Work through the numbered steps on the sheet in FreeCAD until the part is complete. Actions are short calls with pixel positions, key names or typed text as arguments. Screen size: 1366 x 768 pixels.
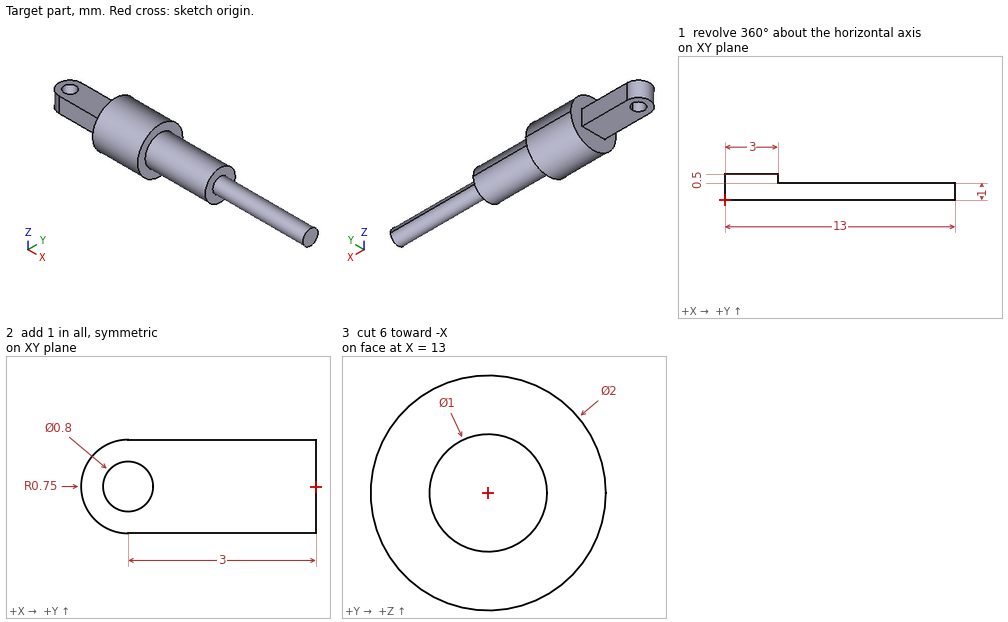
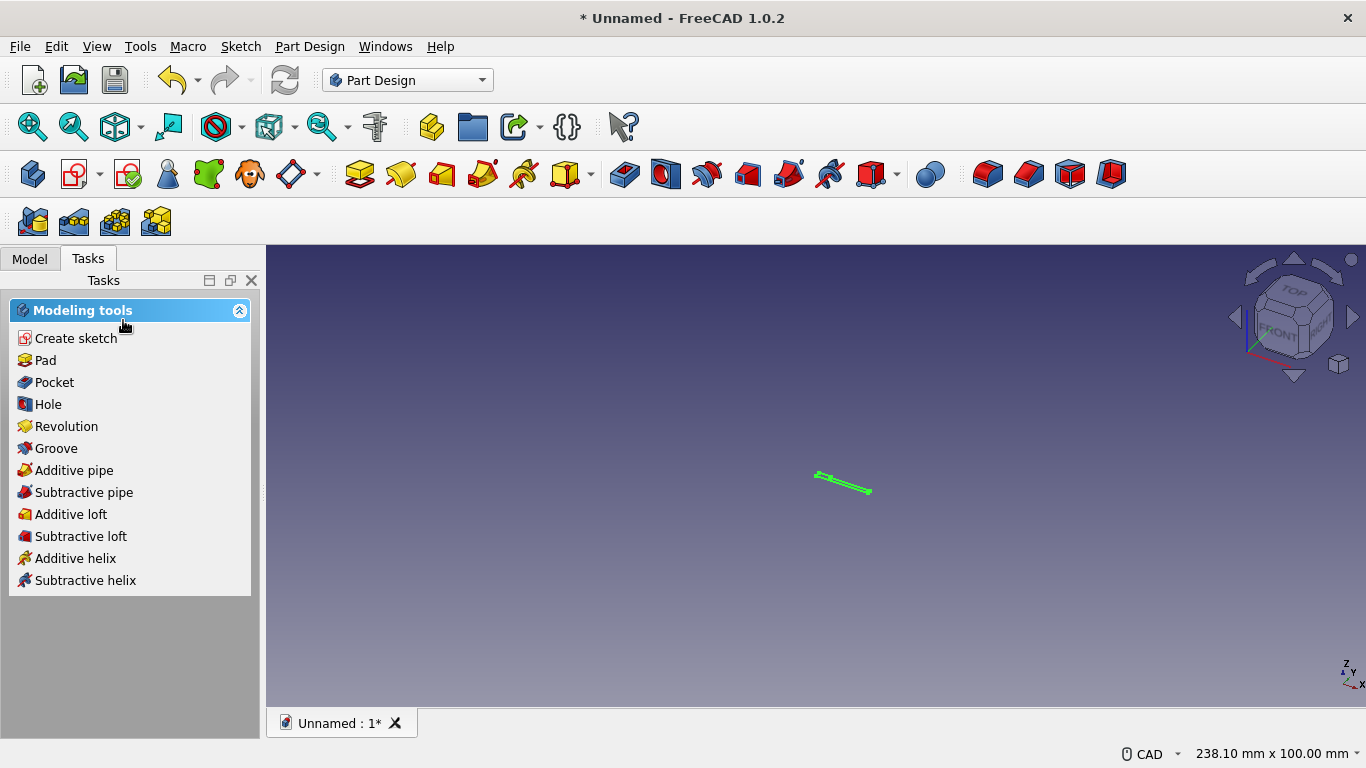
click(401, 174)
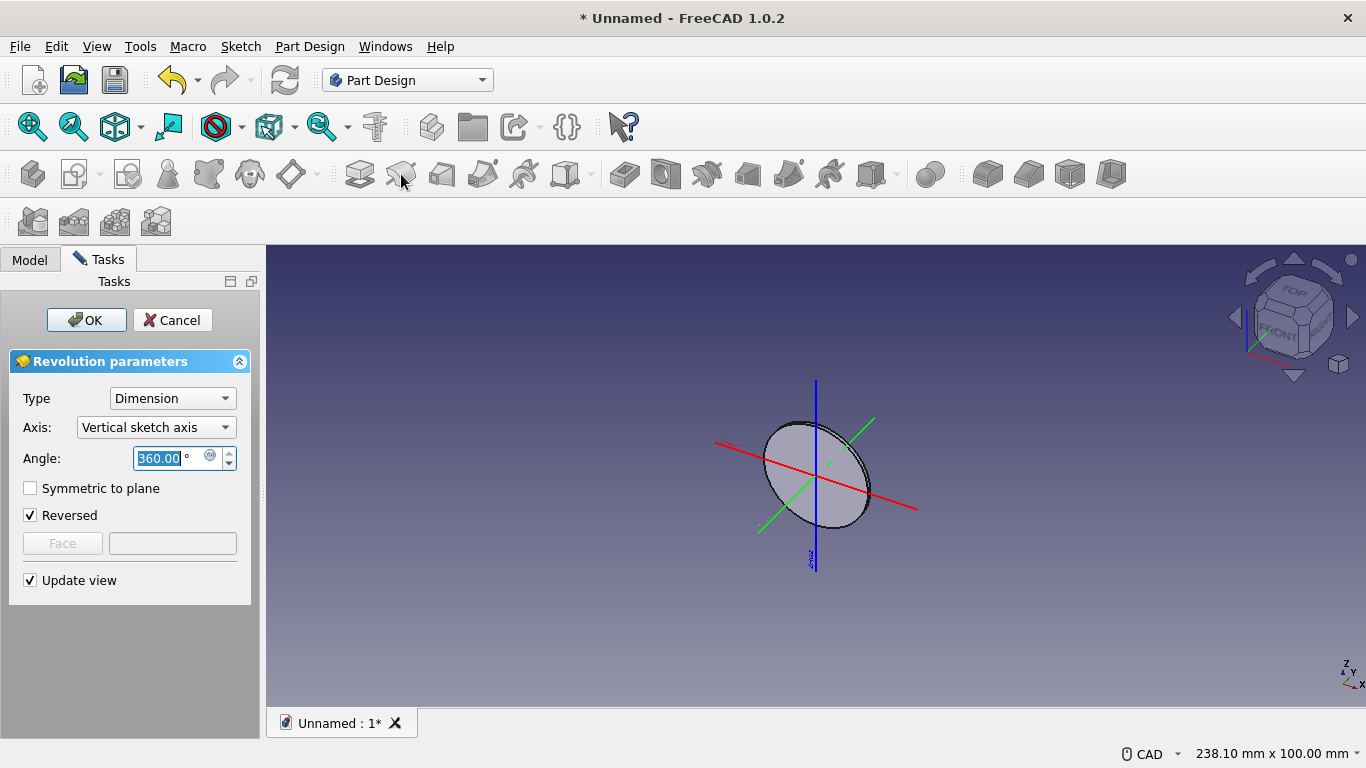
click(157, 428)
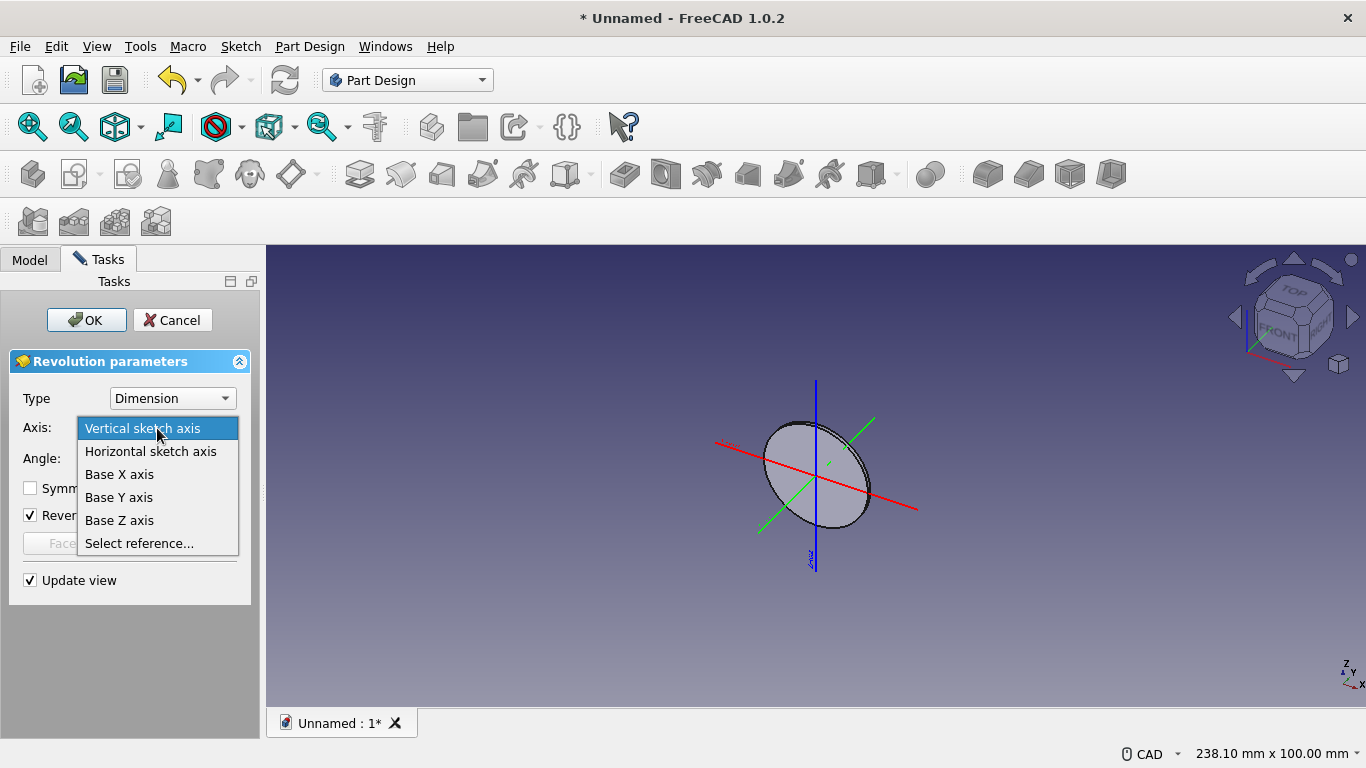
click(156, 452)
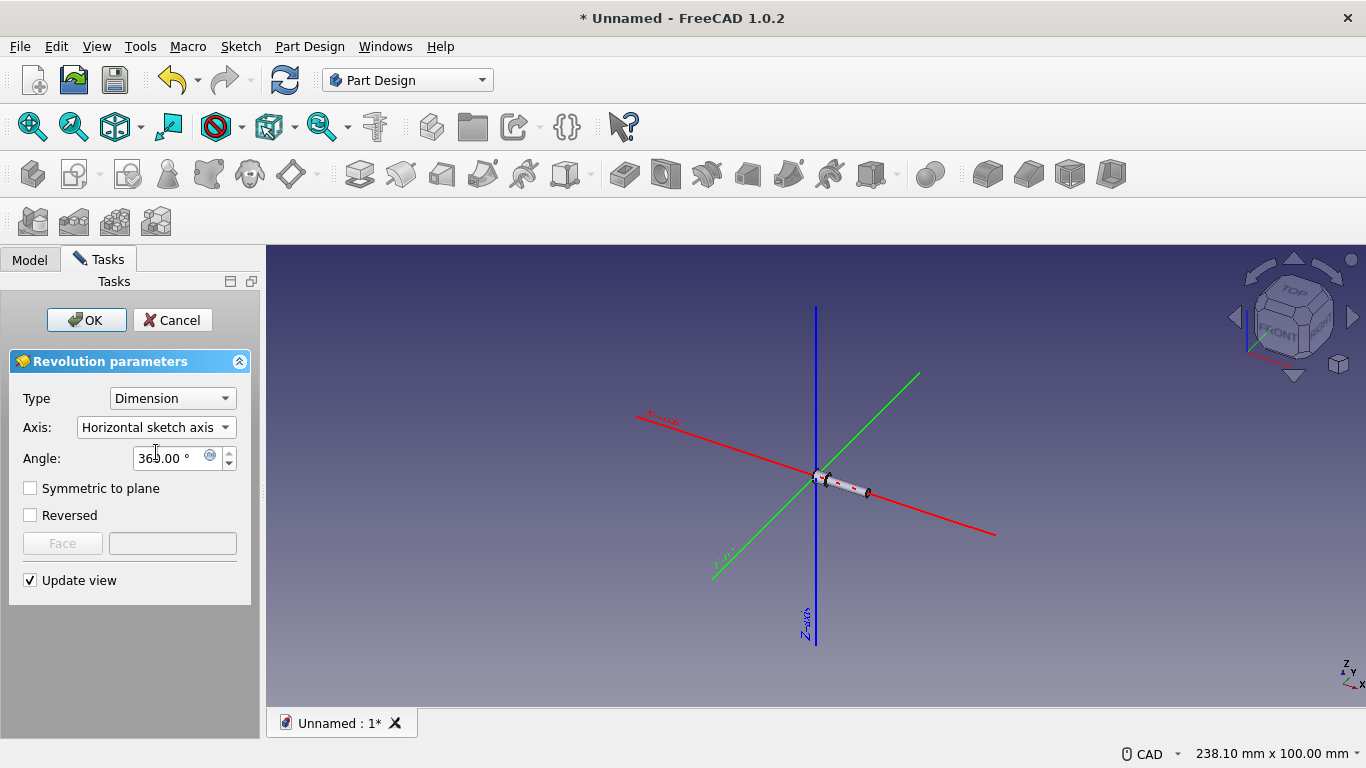
click(87, 320)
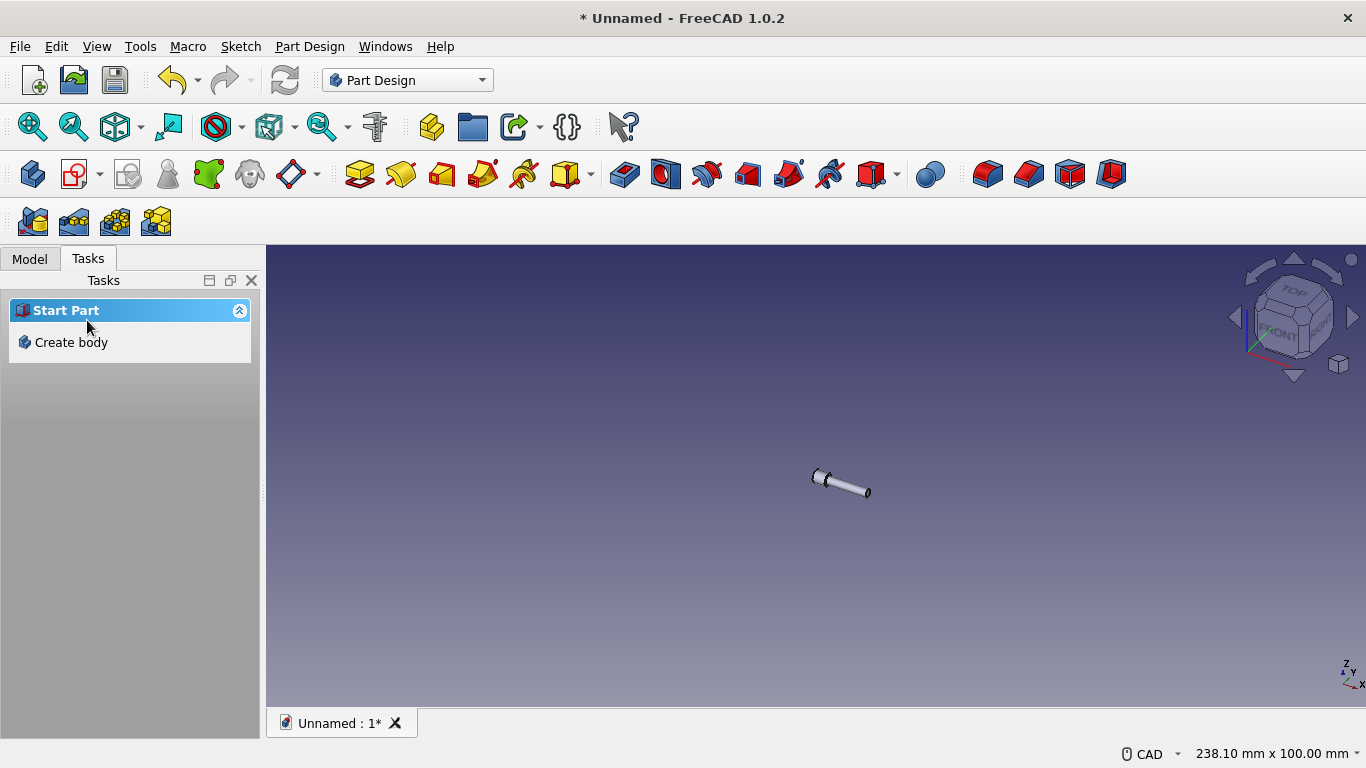
click(33, 128)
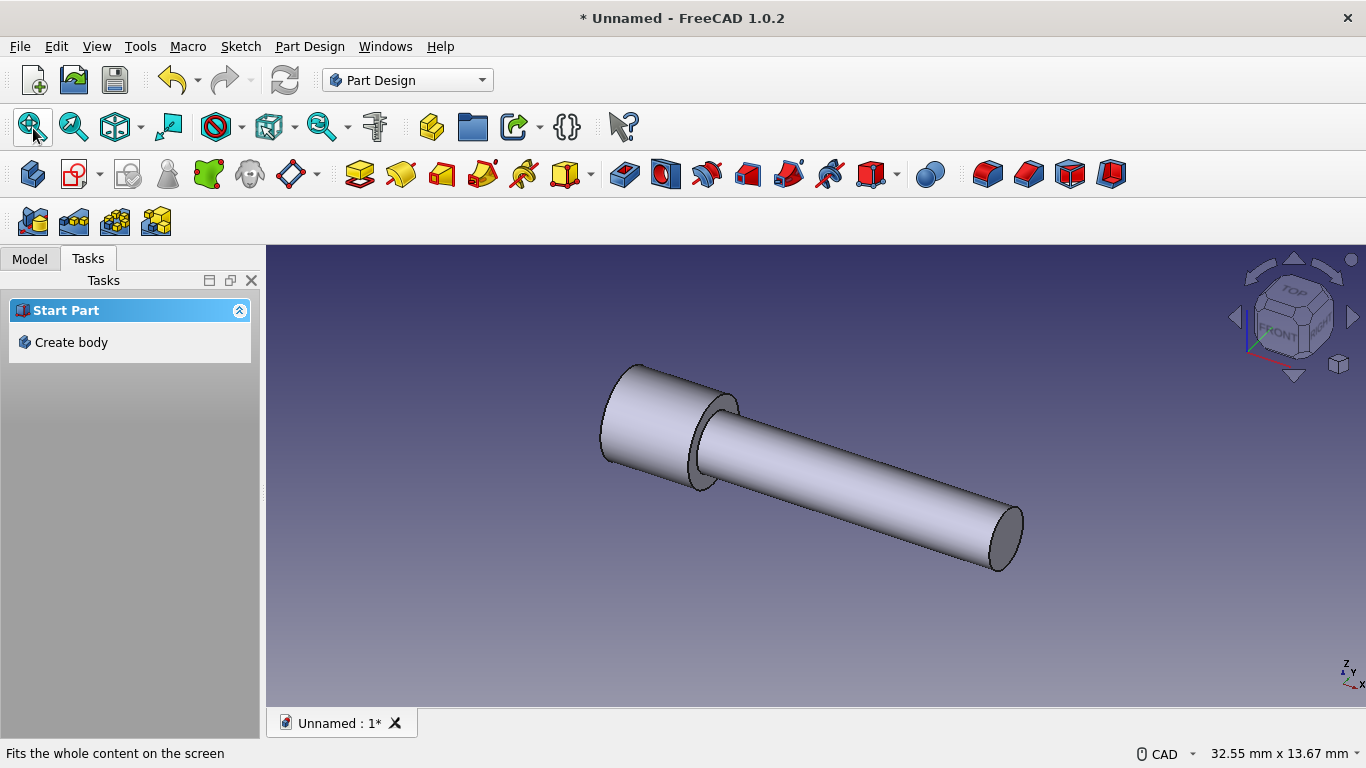
click(74, 174)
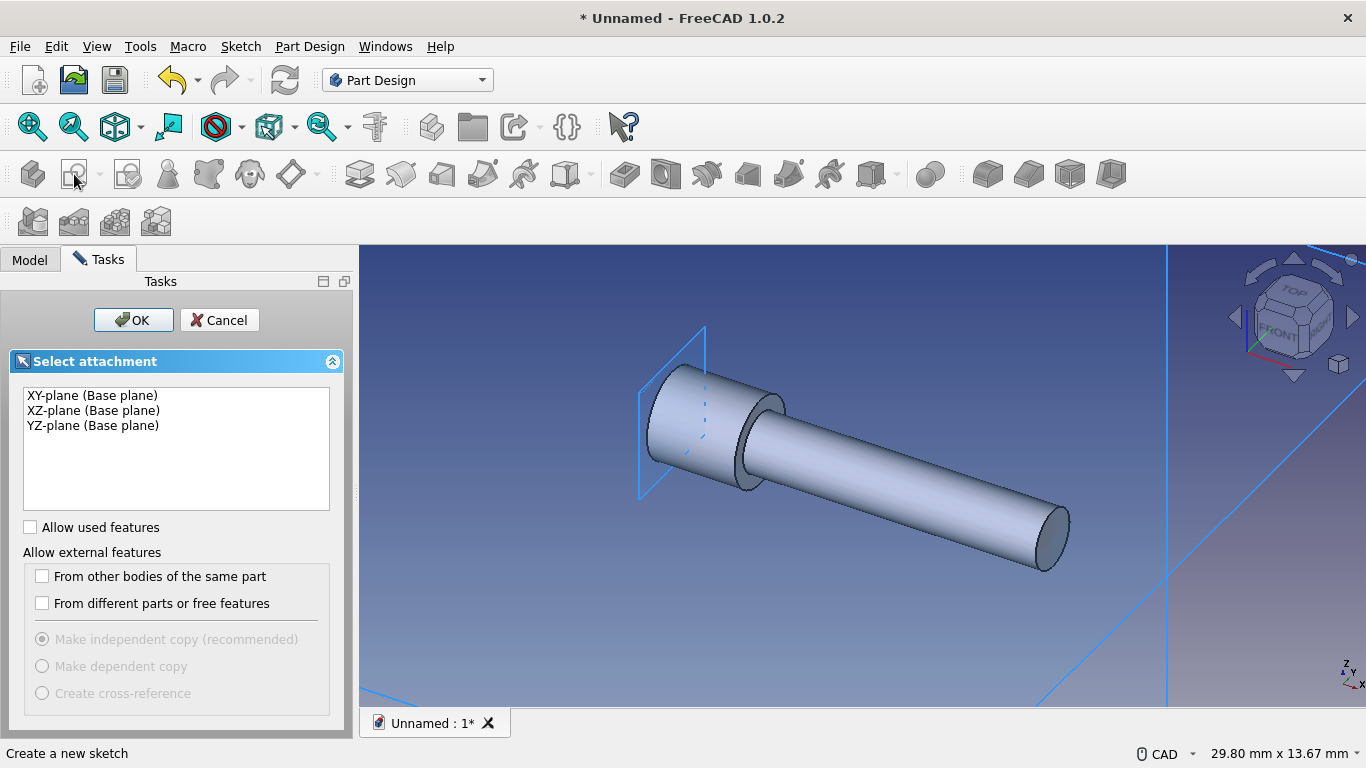
click(84, 396)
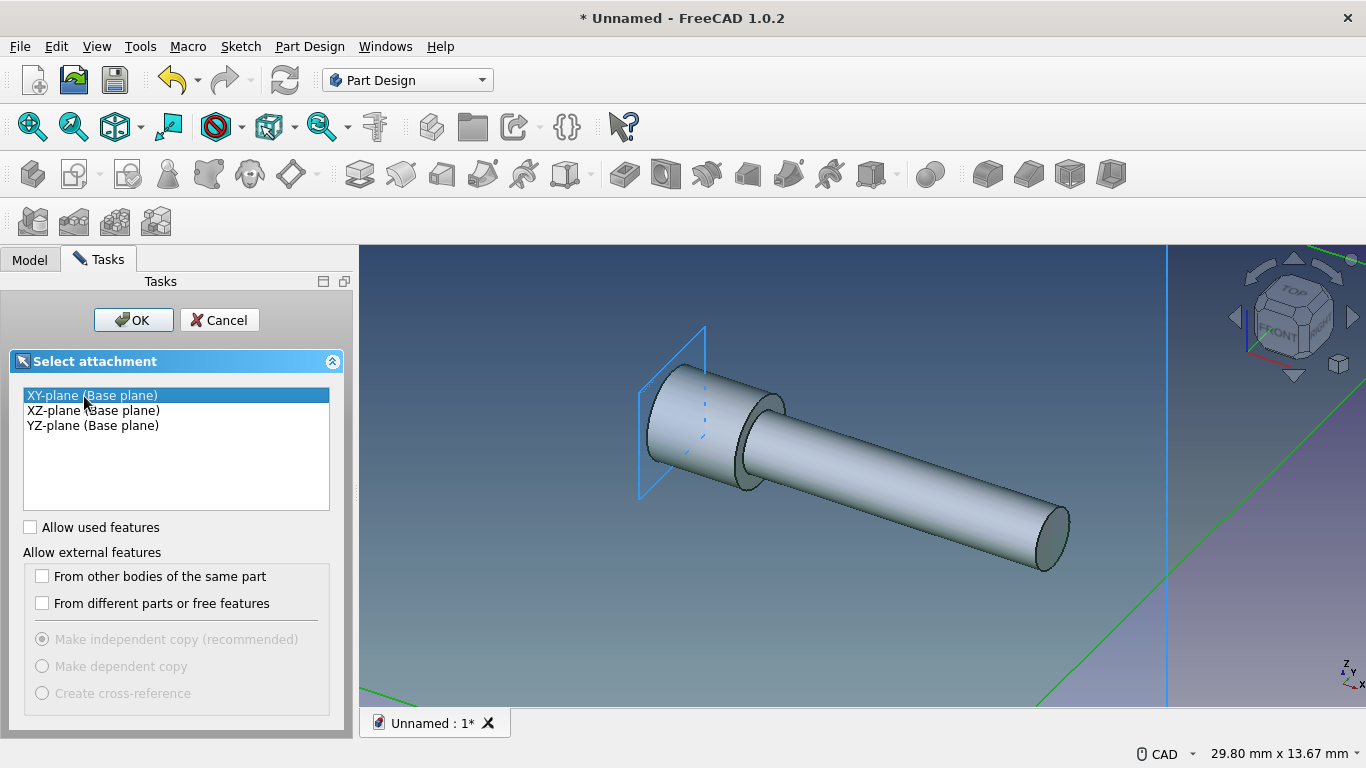
click(134, 320)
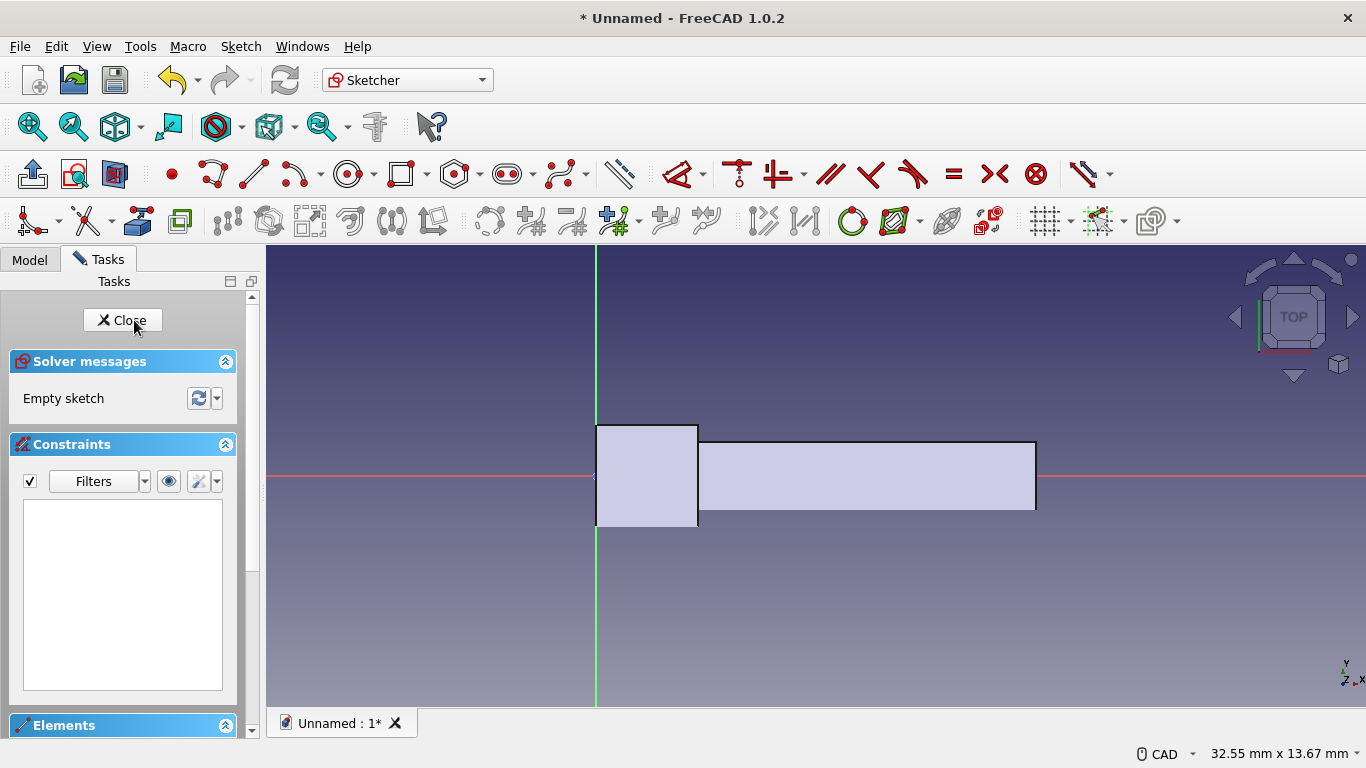
key(q)
key(s)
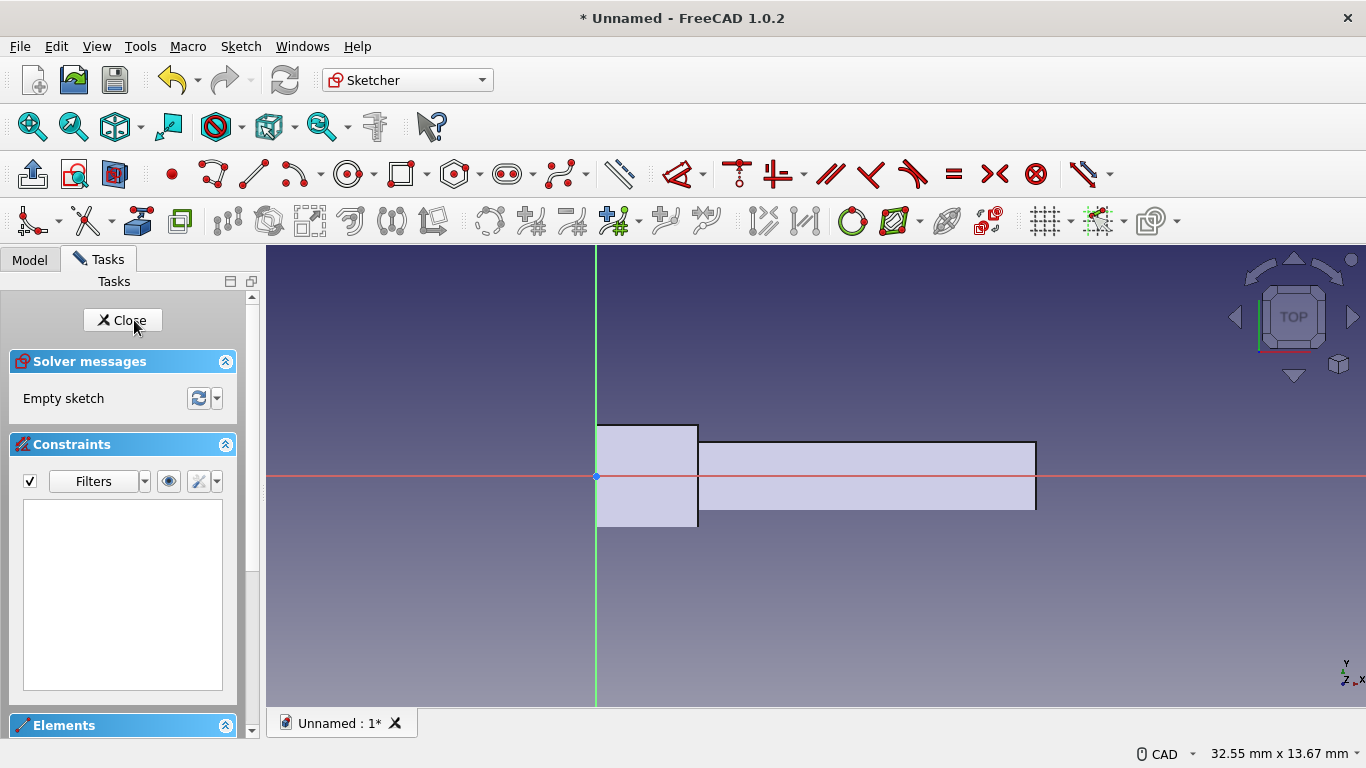
scroll(479, 476, up, 8)